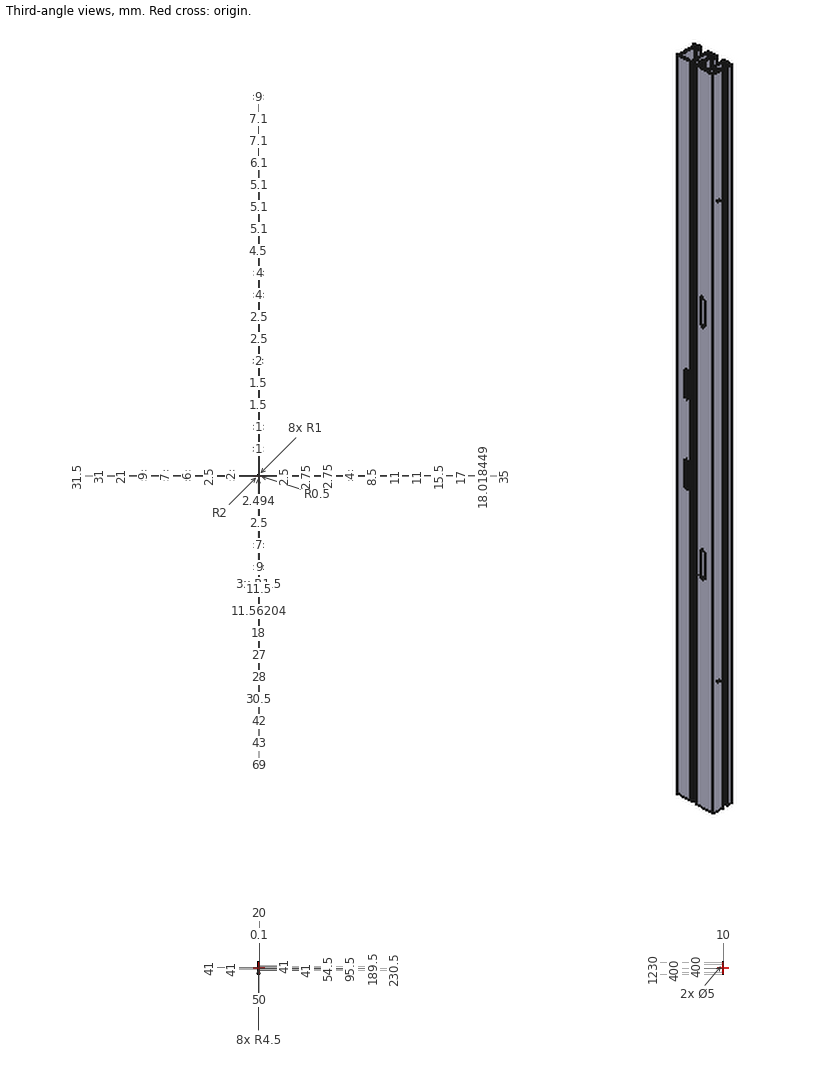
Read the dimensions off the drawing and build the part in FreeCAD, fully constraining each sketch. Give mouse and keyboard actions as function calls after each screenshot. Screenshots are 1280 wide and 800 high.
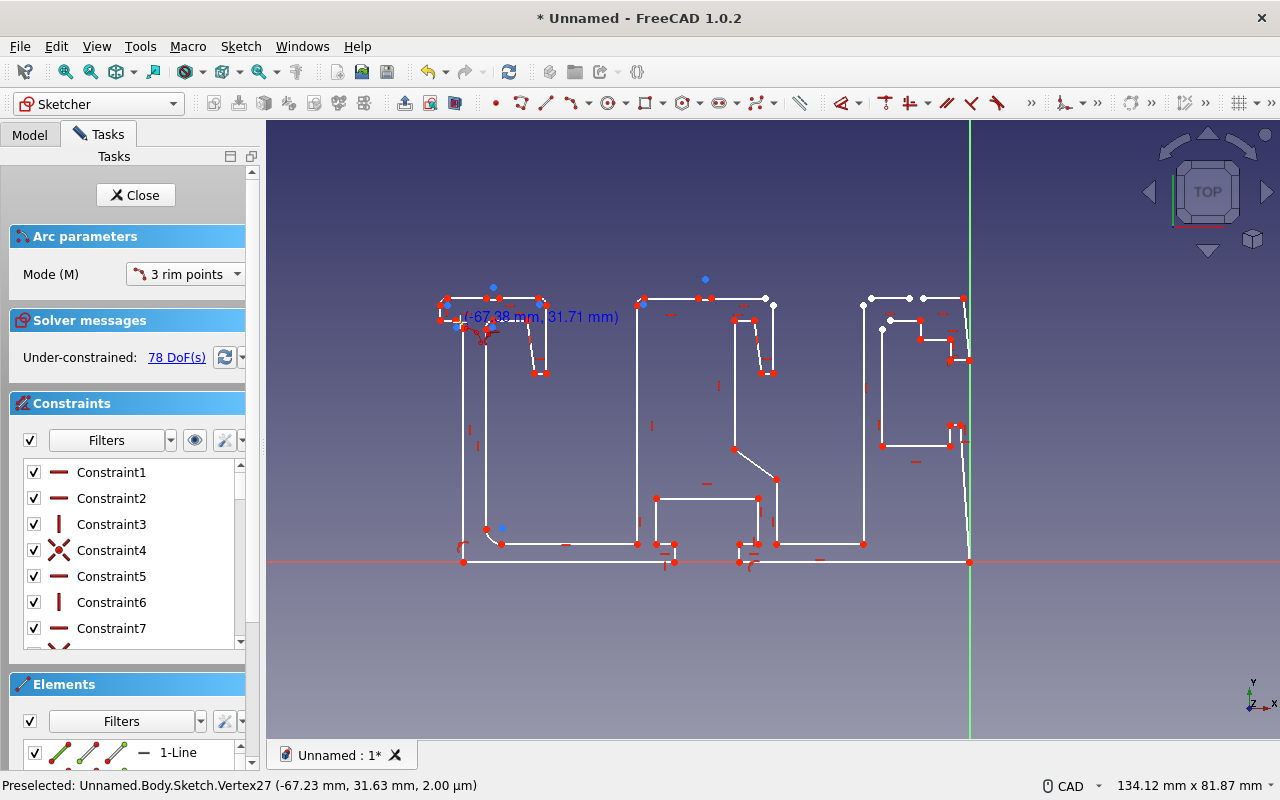
scroll(883, 328, up, 2)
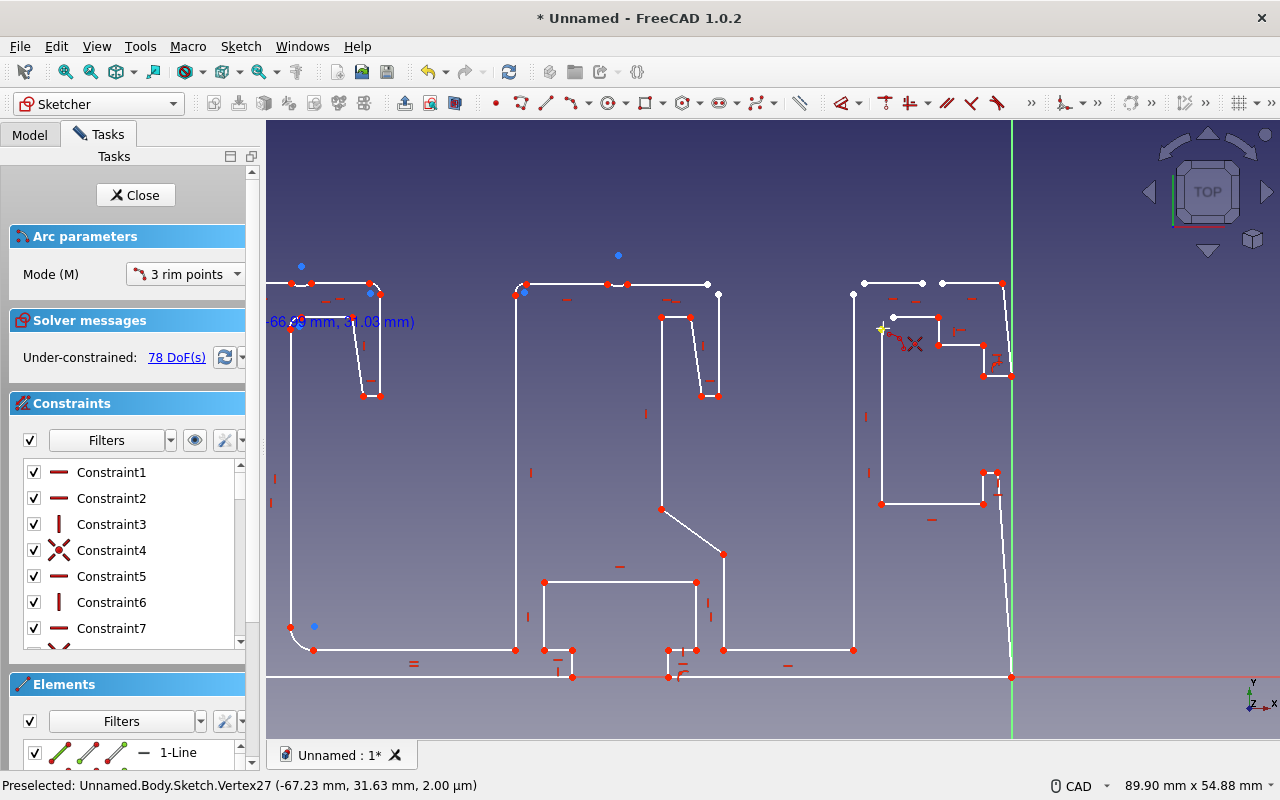
click(882, 330)
click(894, 317)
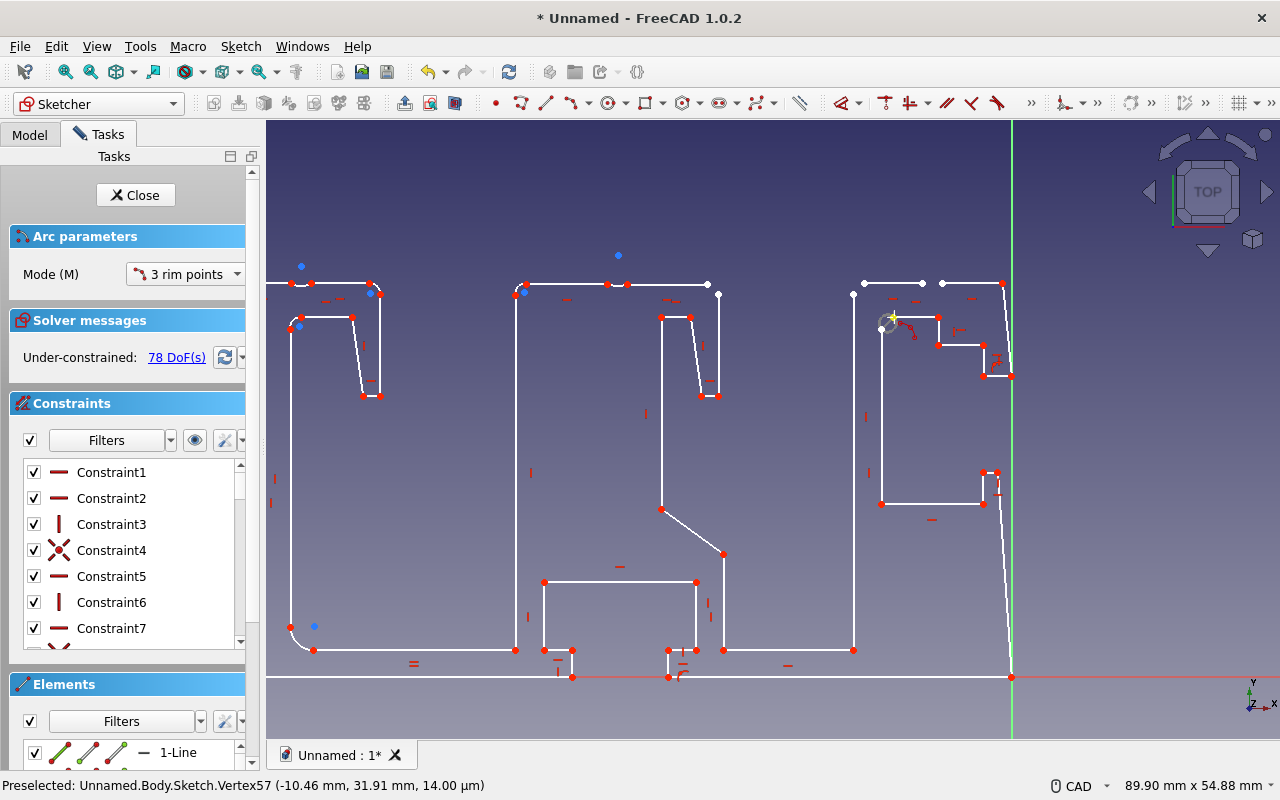
scroll(885, 320, up, 8)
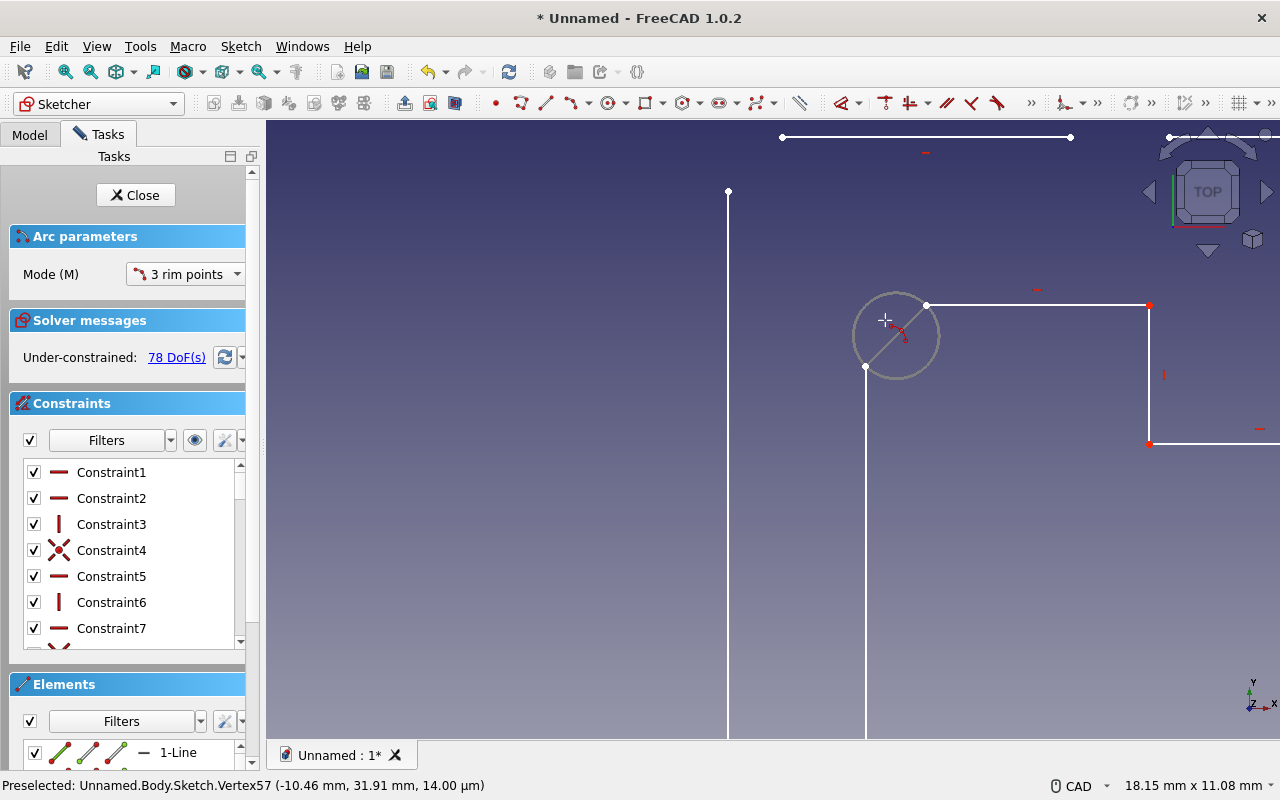
click(885, 317)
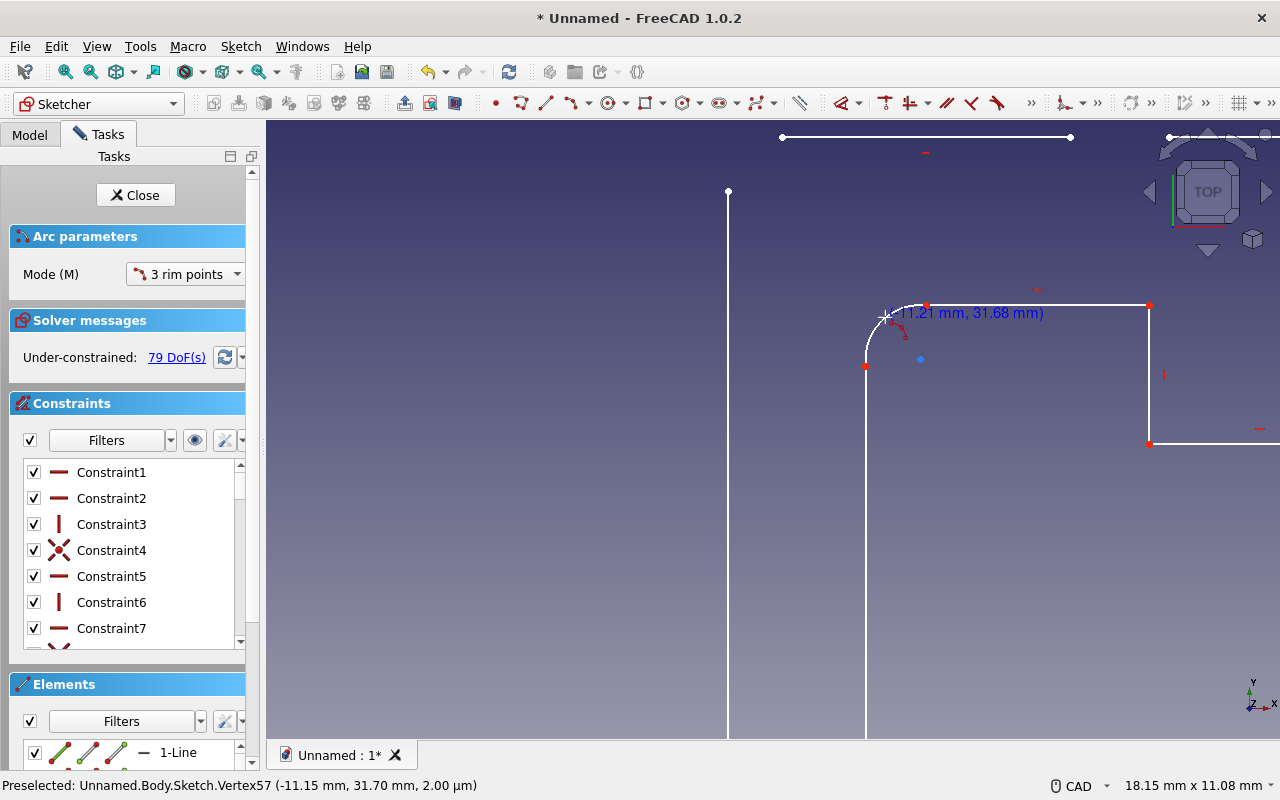
scroll(884, 323, down, 10)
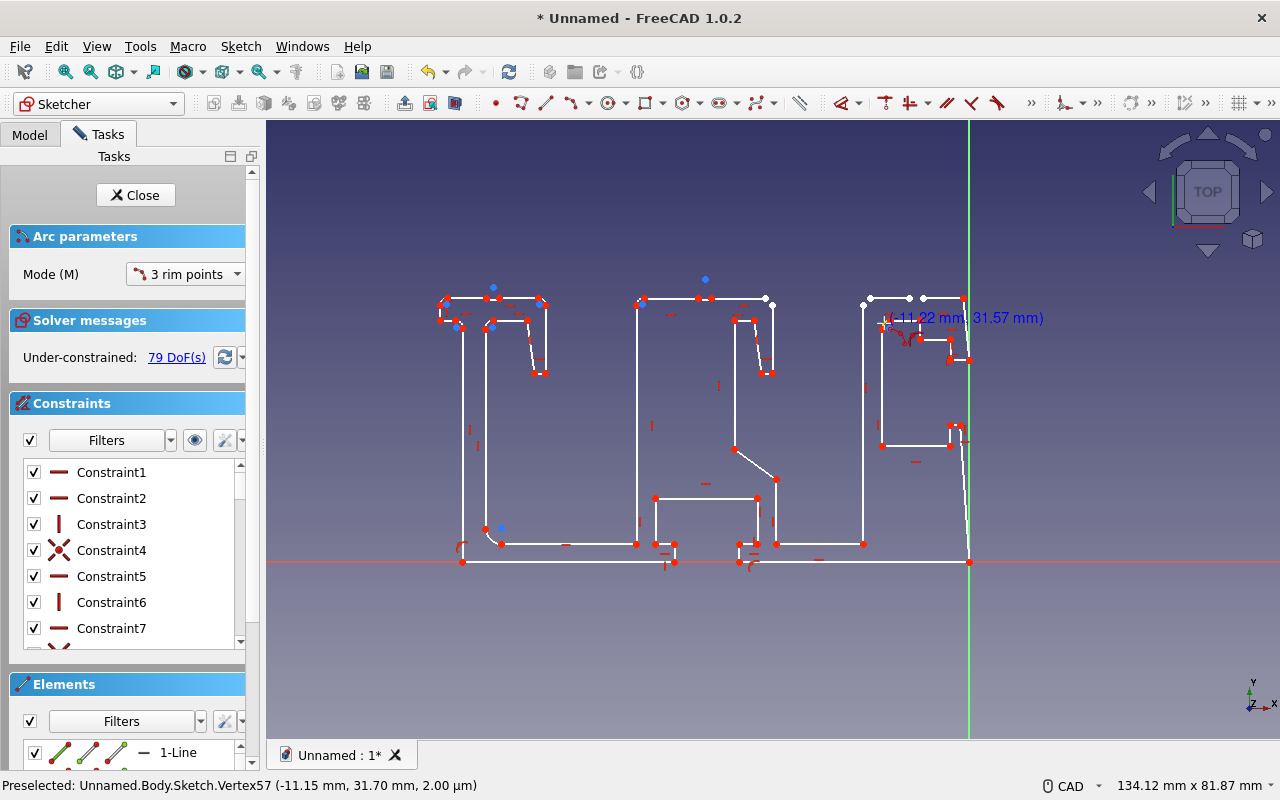
click(923, 298)
click(910, 298)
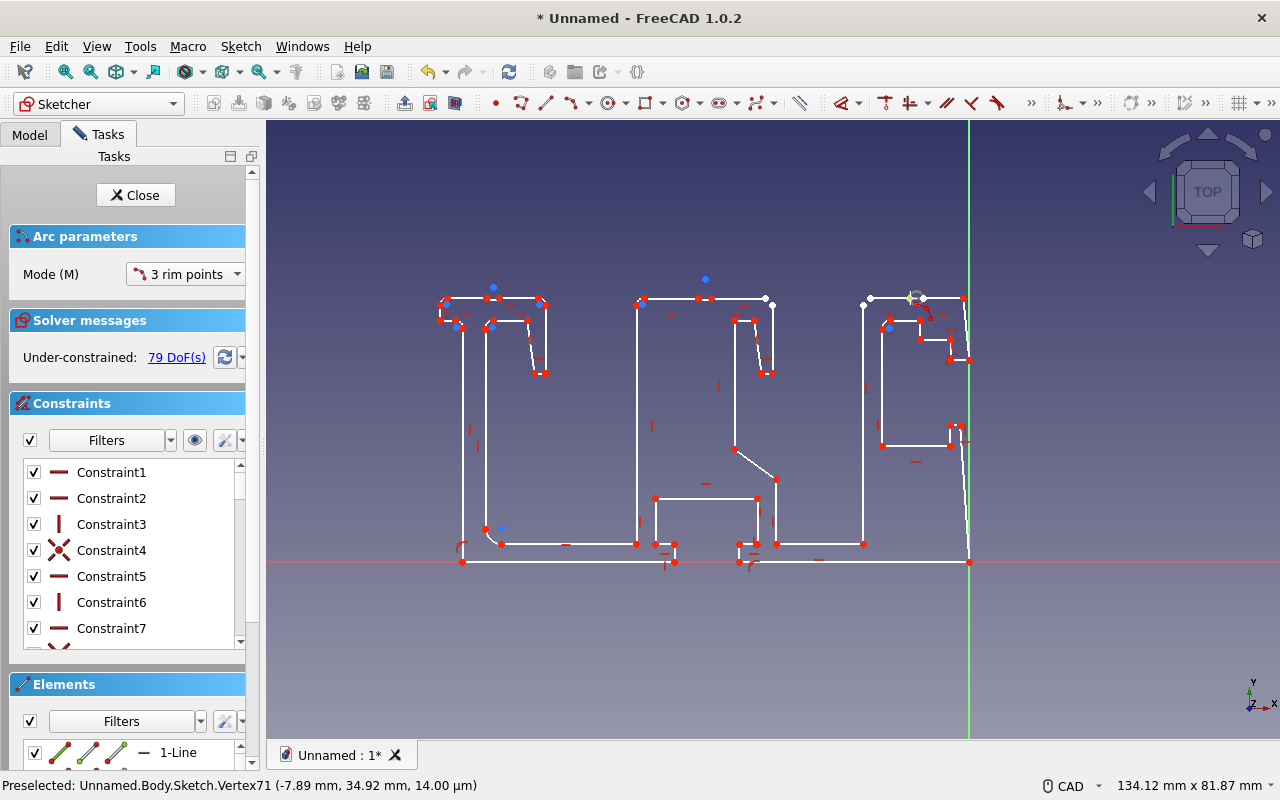
scroll(916, 300, up, 10)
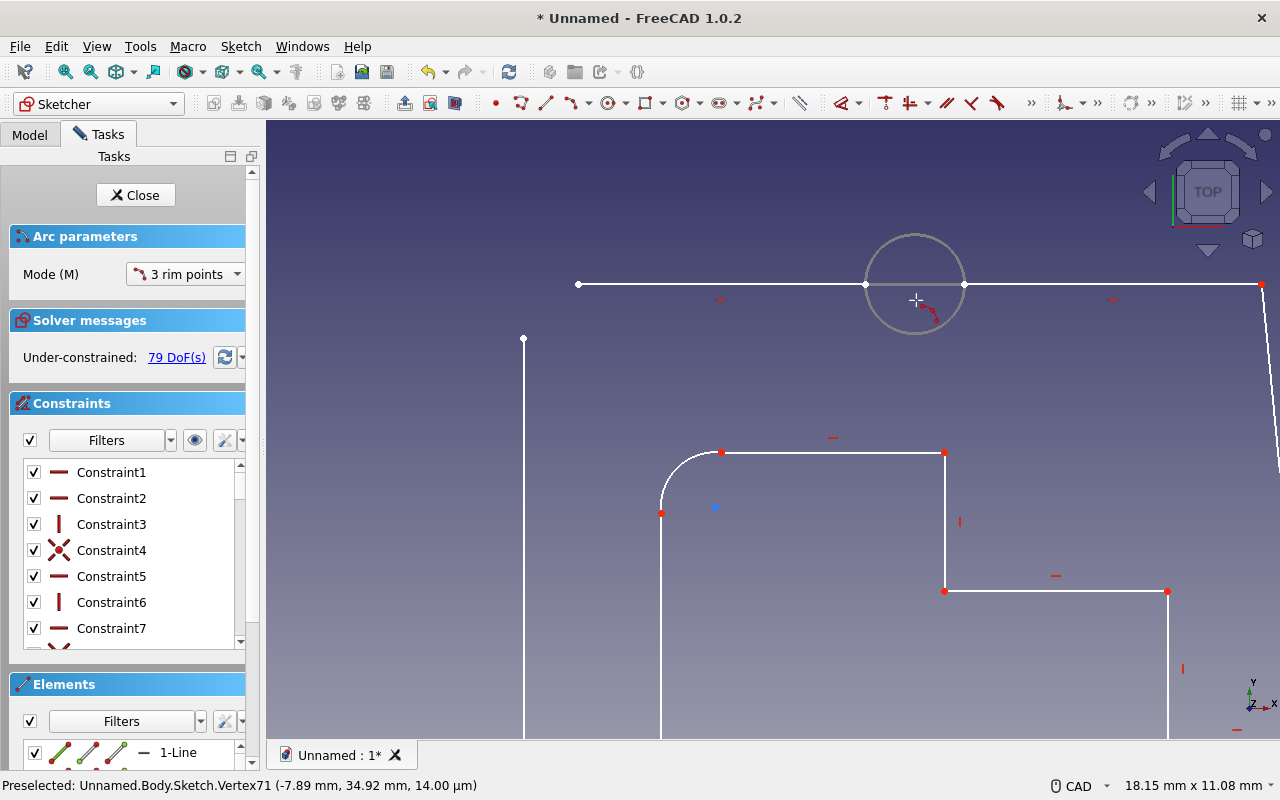
click(915, 297)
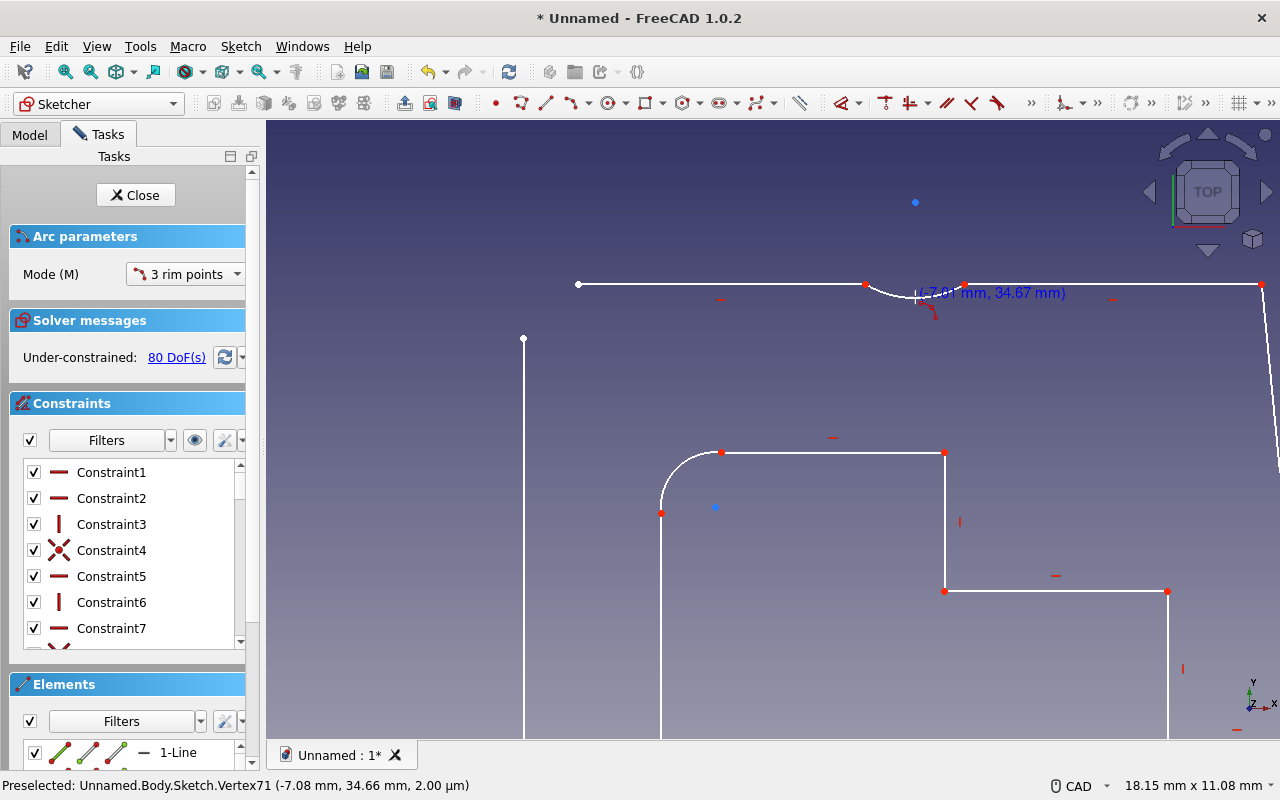
scroll(916, 300, down, 10)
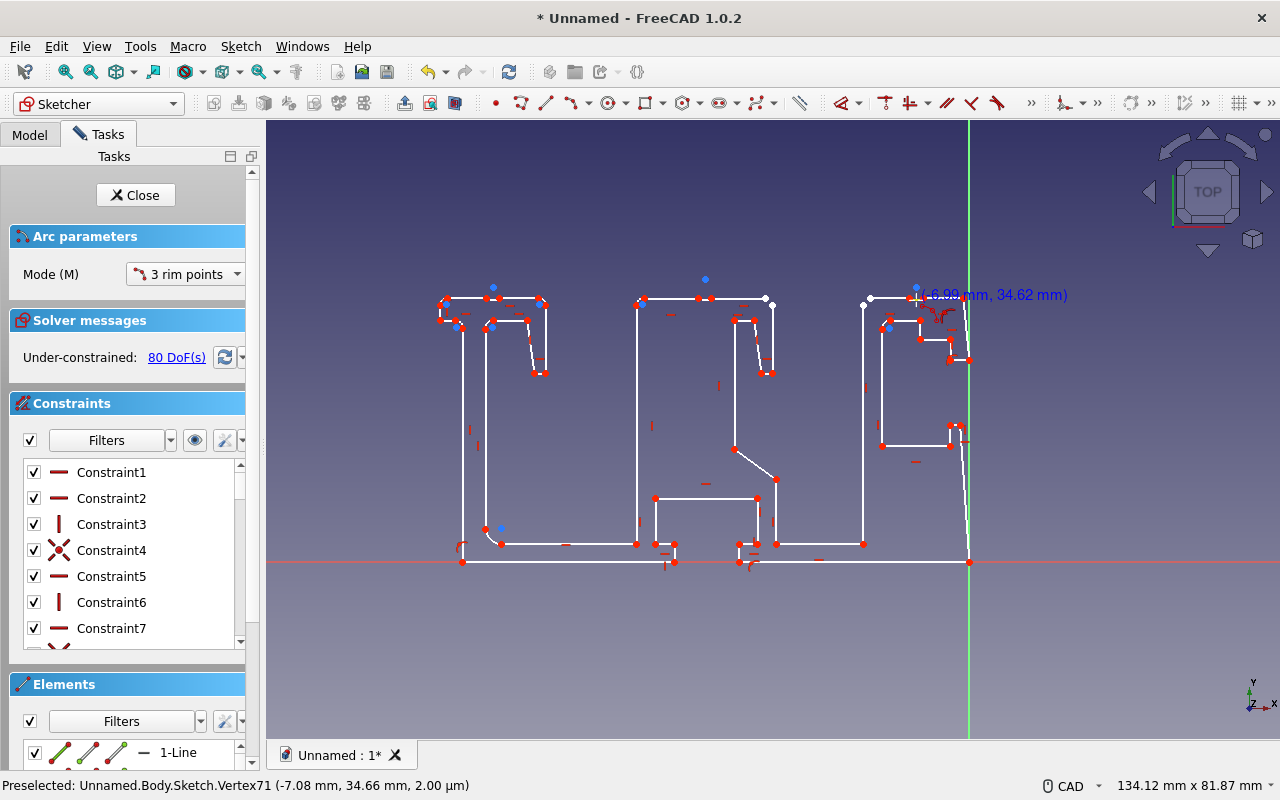
scroll(871, 298, up, 2)